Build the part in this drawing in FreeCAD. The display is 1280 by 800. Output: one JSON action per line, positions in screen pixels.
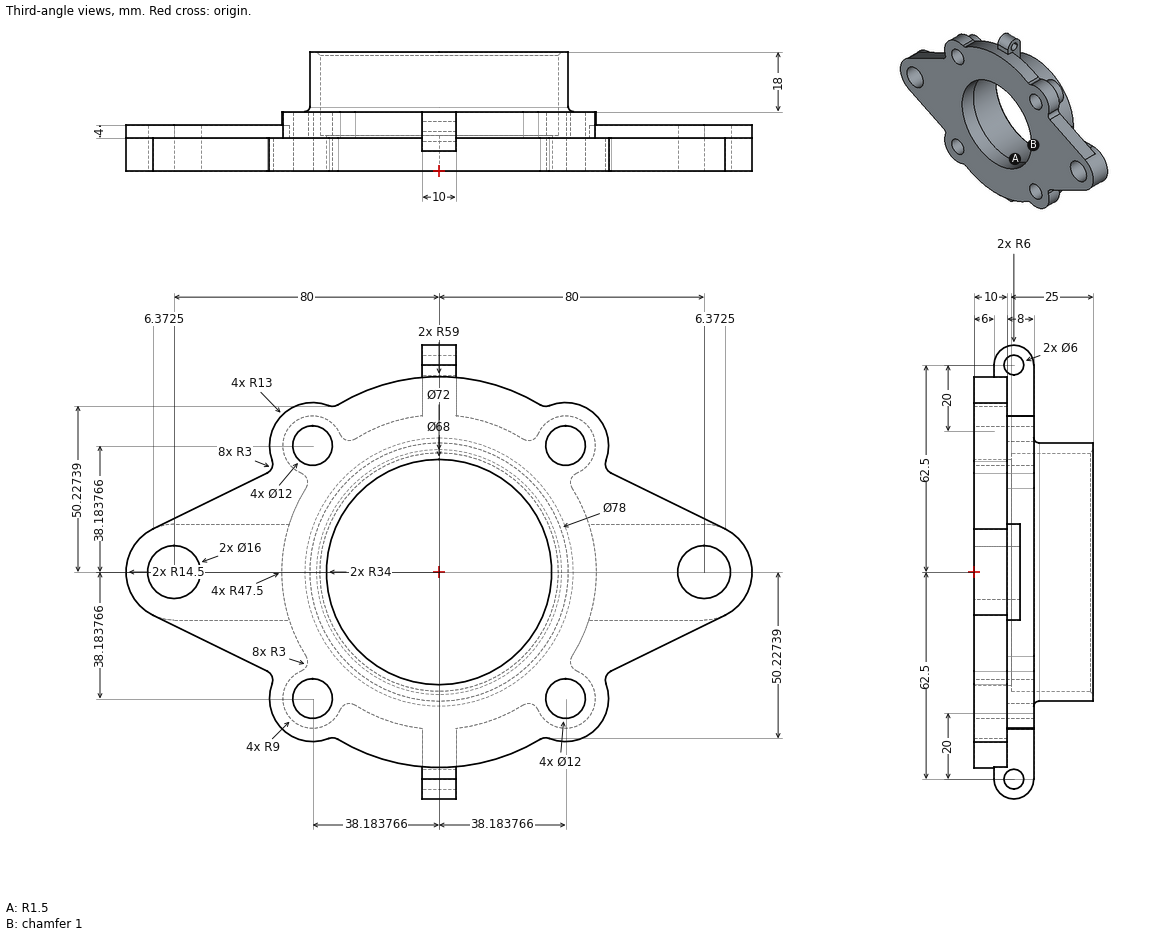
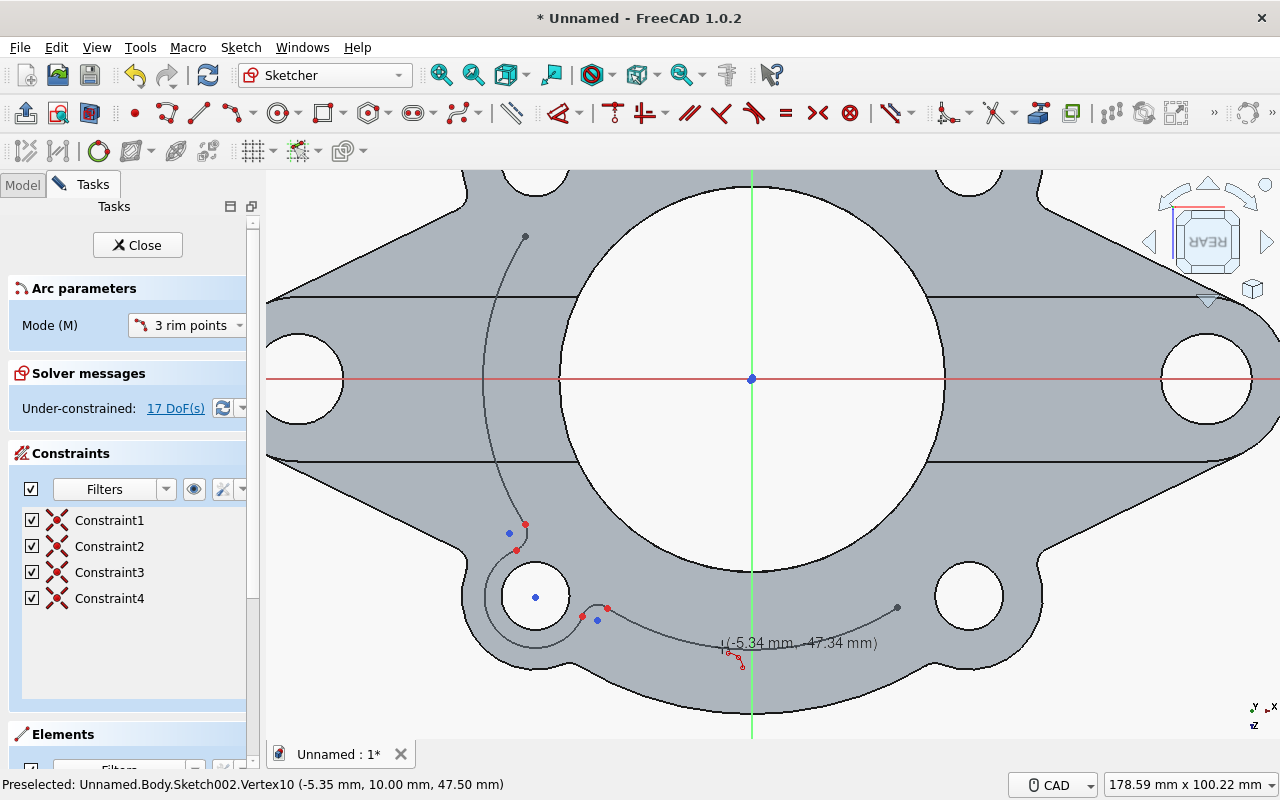
{"action": "left_click", "coordinate": [897, 608]}
{"action": "left_click", "coordinate": [922, 615]}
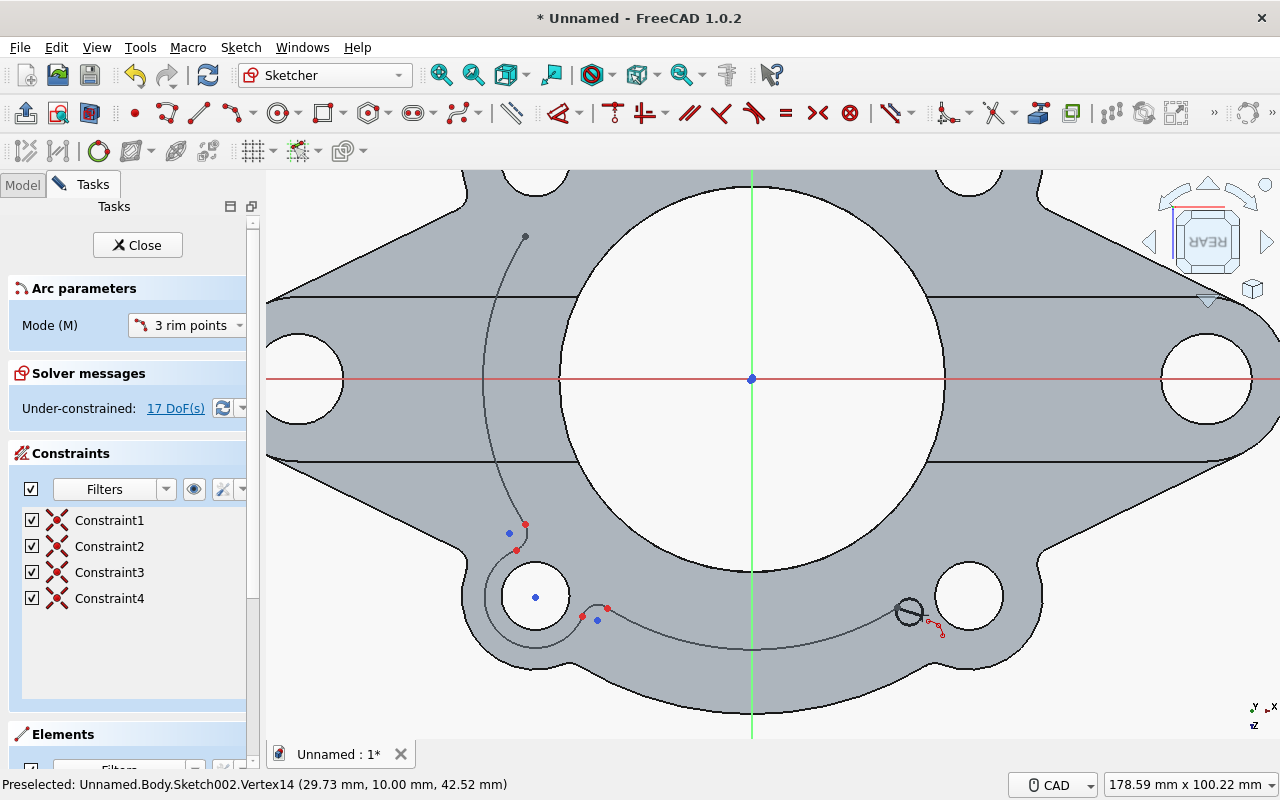
{"action": "scroll", "coordinate": [911, 605], "scroll_direction": "up", "scroll_amount": 5}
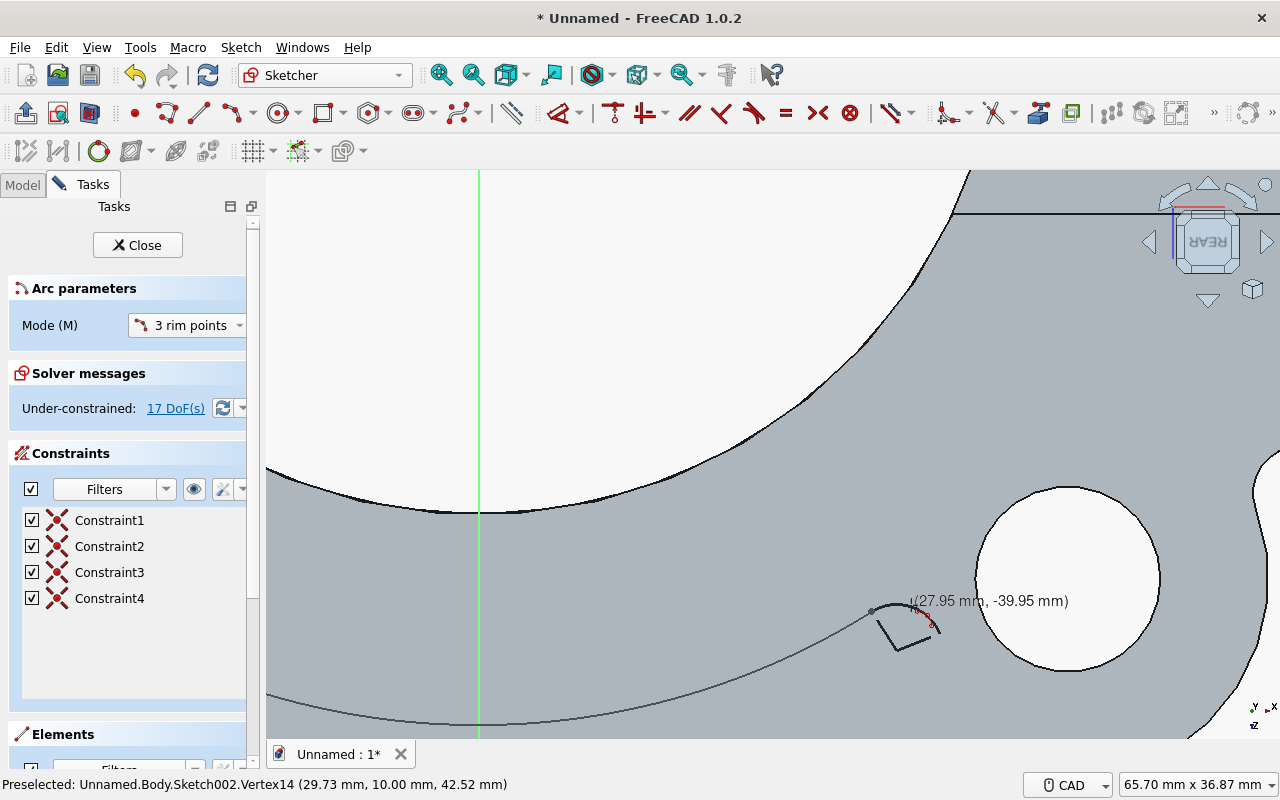
{"action": "left_click", "coordinate": [910, 604]}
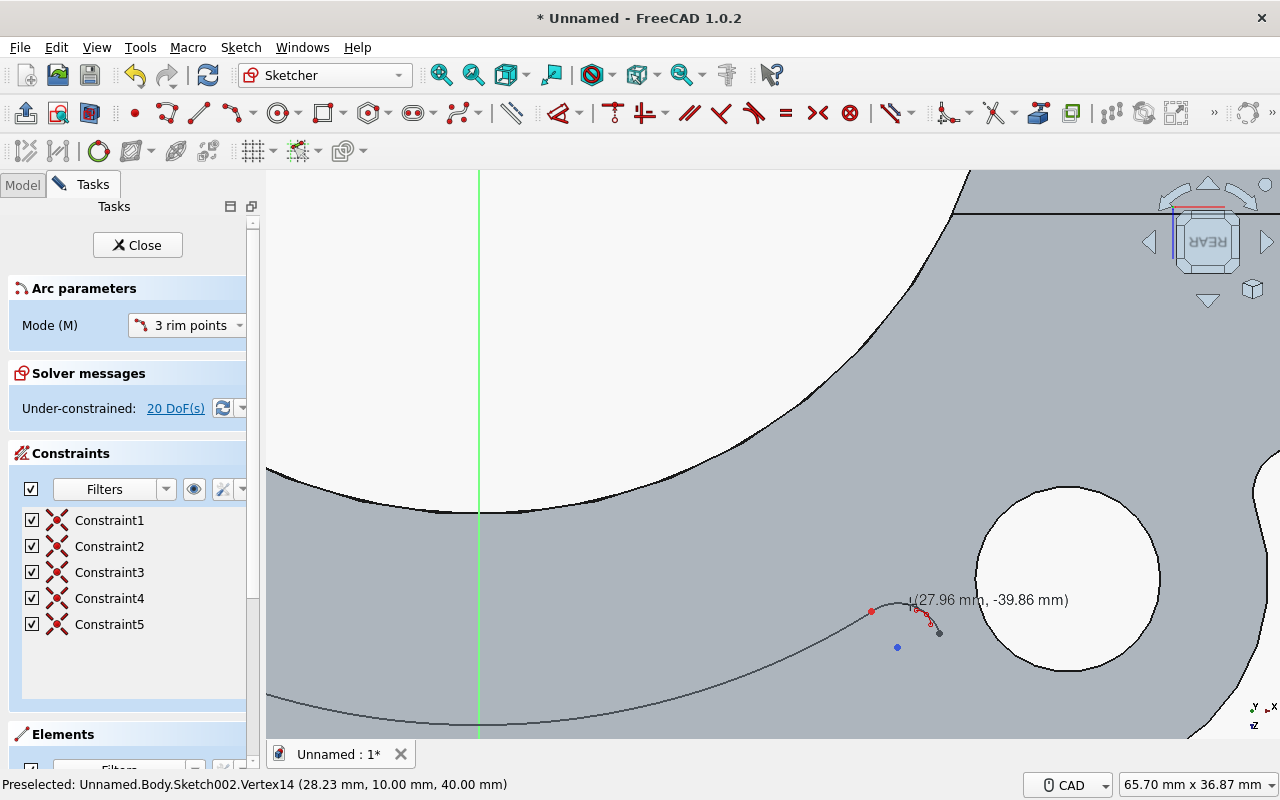
{"action": "scroll", "coordinate": [778, 607], "scroll_direction": "down", "scroll_amount": 7}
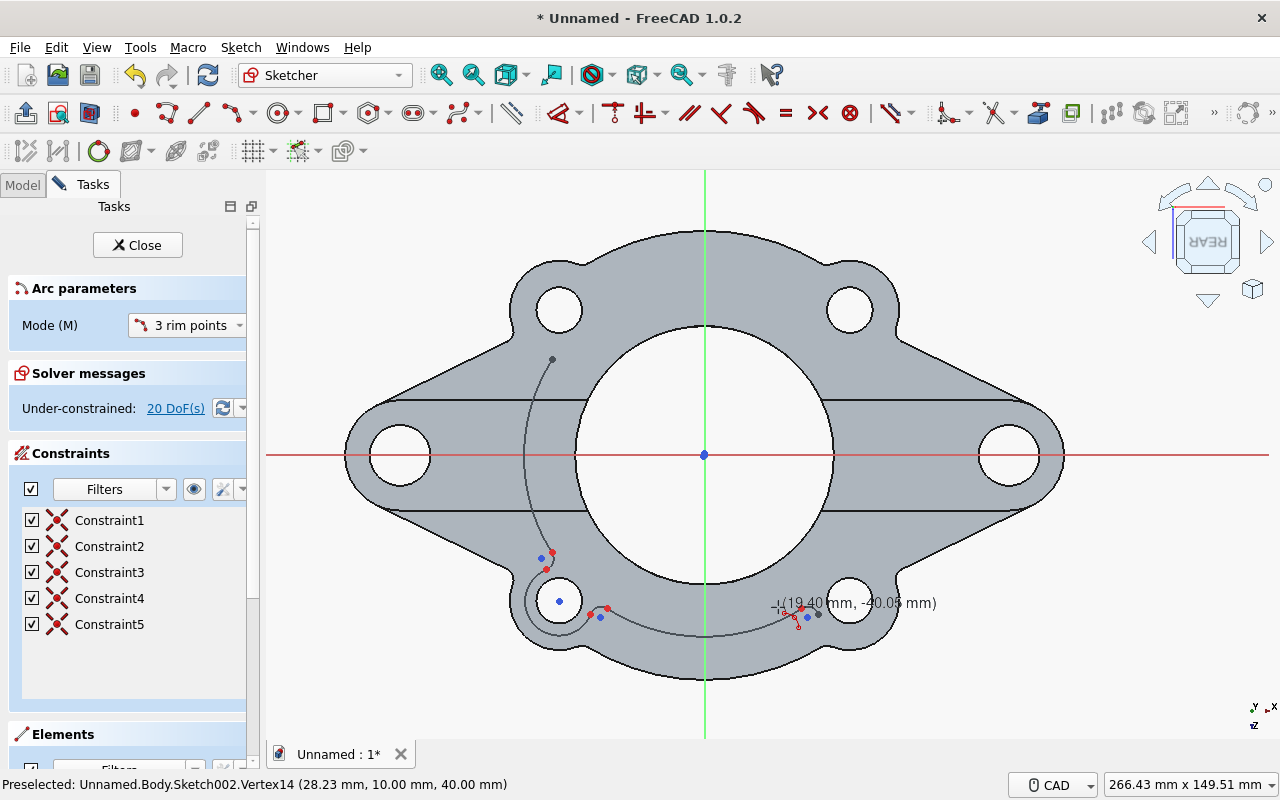
{"action": "scroll", "coordinate": [818, 613], "scroll_direction": "up", "scroll_amount": 2}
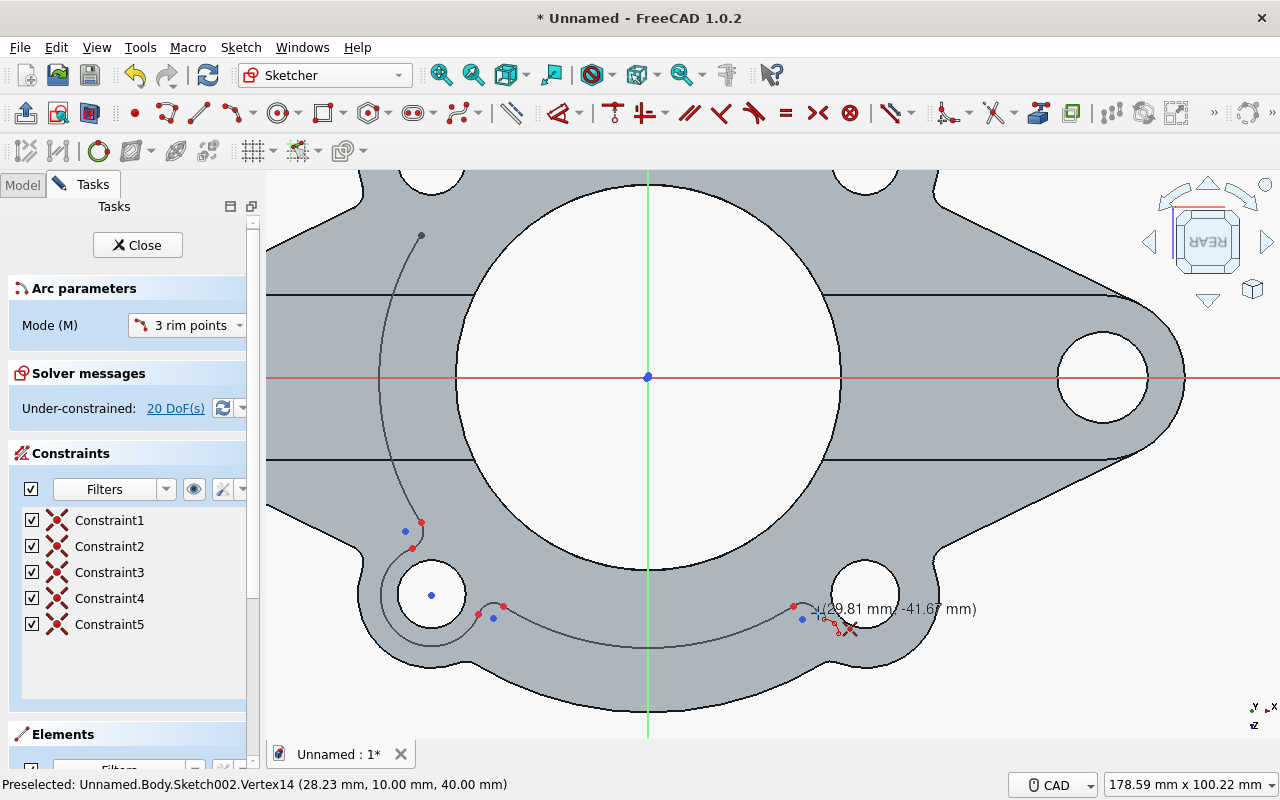
{"action": "left_click", "coordinate": [818, 614]}
{"action": "left_click", "coordinate": [884, 547]}
{"action": "left_click", "coordinate": [901, 630]}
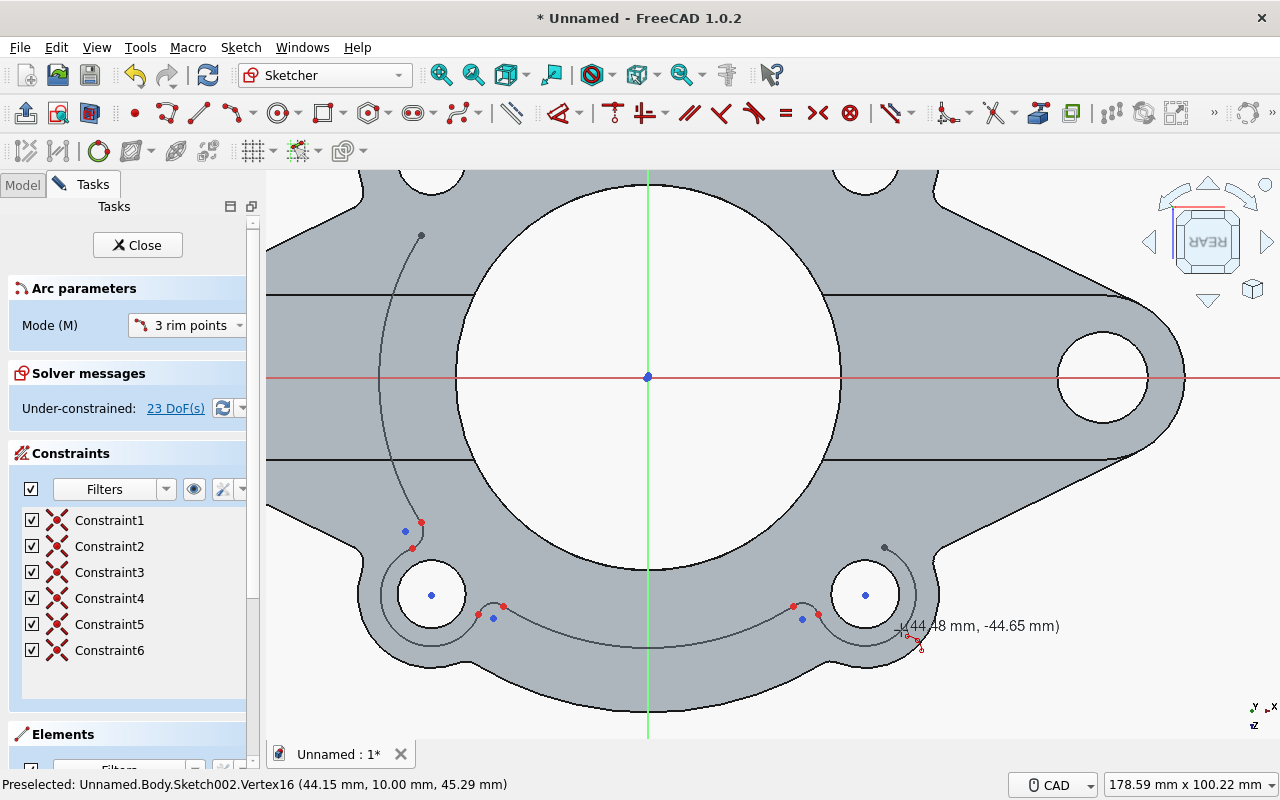
{"action": "left_click", "coordinate": [884, 548]}
{"action": "left_click", "coordinate": [876, 522]}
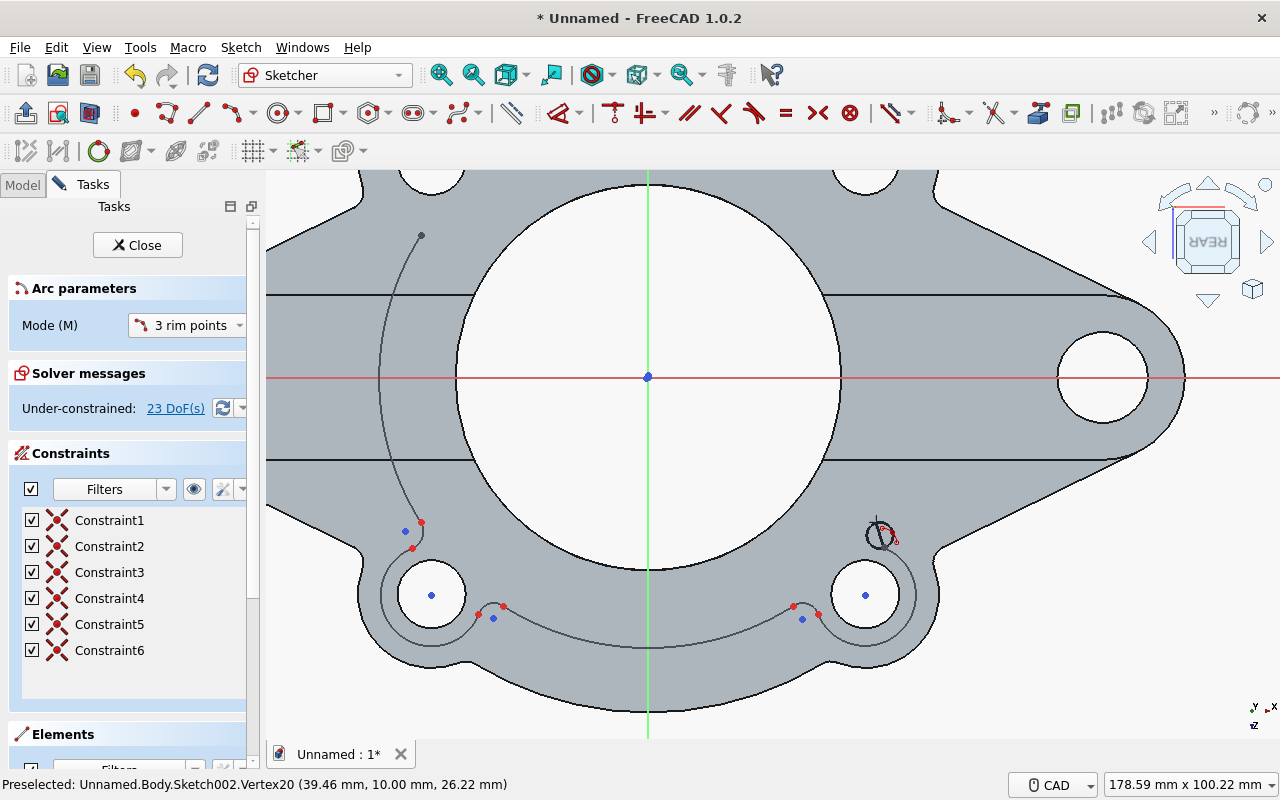
{"action": "scroll", "coordinate": [874, 536], "scroll_direction": "up", "scroll_amount": 5}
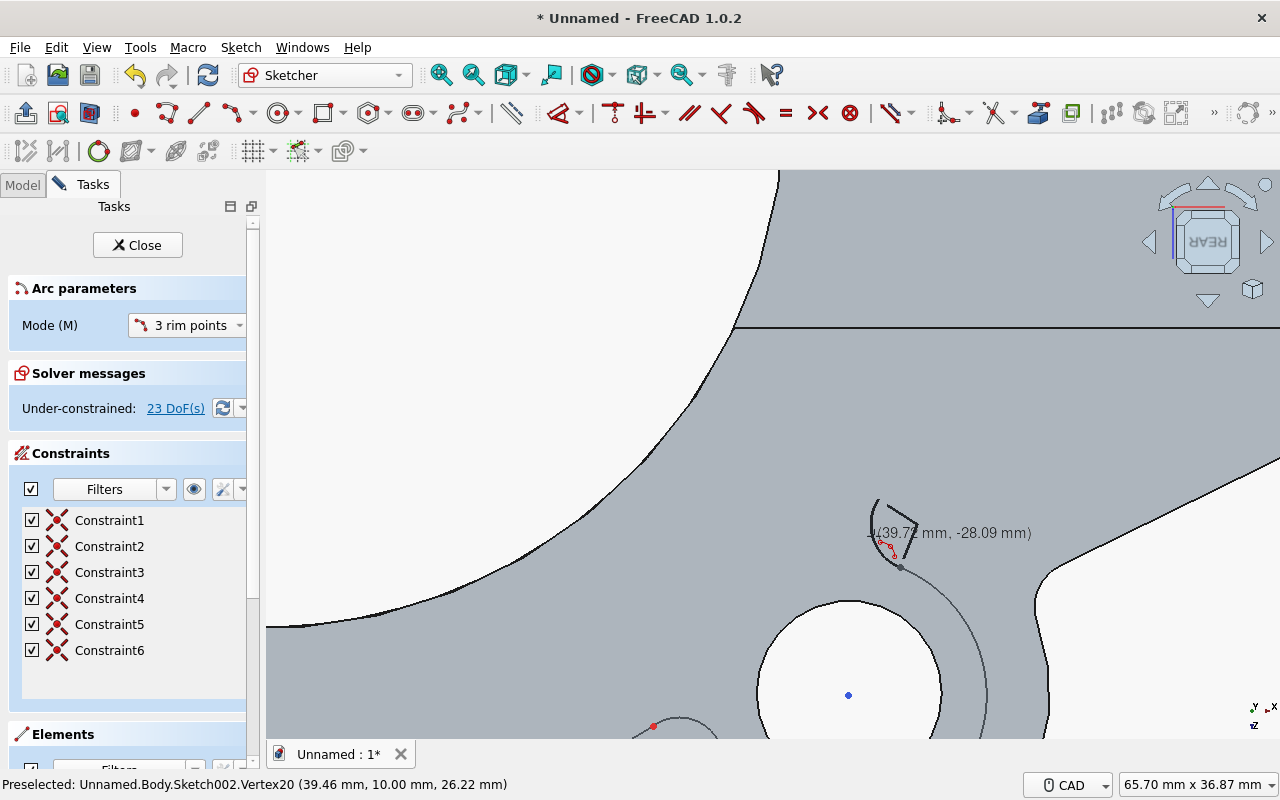
{"action": "left_click", "coordinate": [874, 536]}